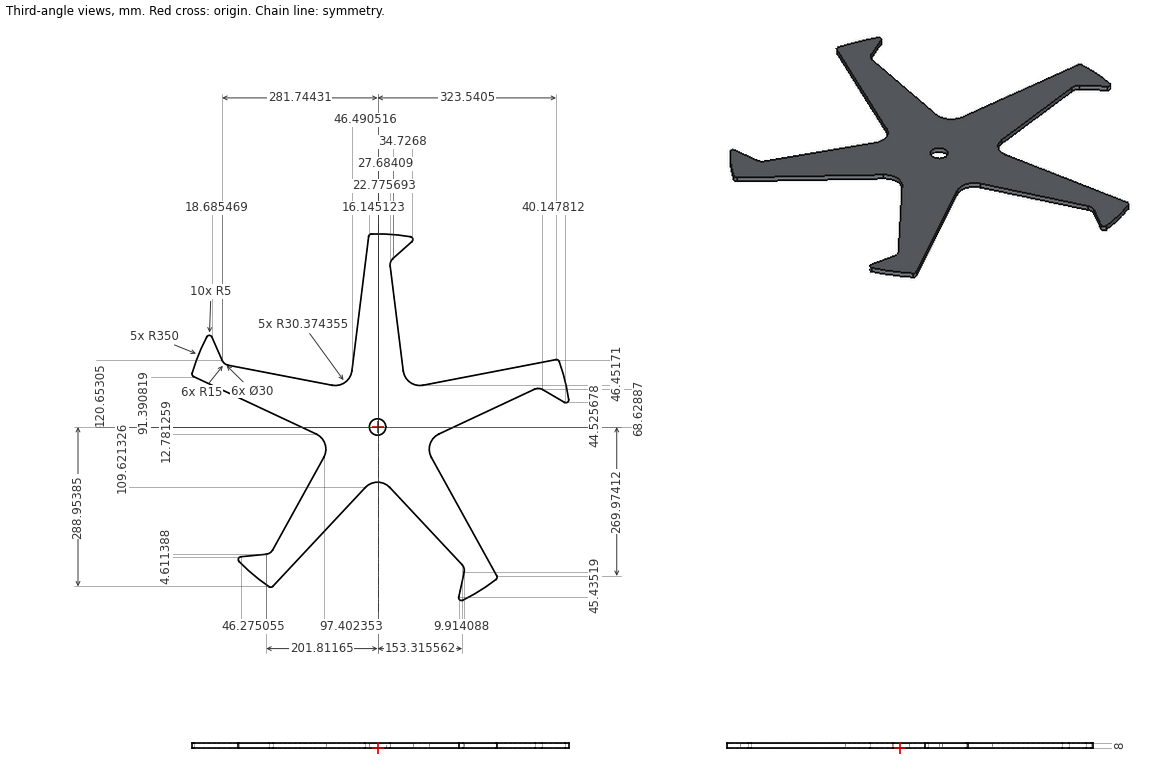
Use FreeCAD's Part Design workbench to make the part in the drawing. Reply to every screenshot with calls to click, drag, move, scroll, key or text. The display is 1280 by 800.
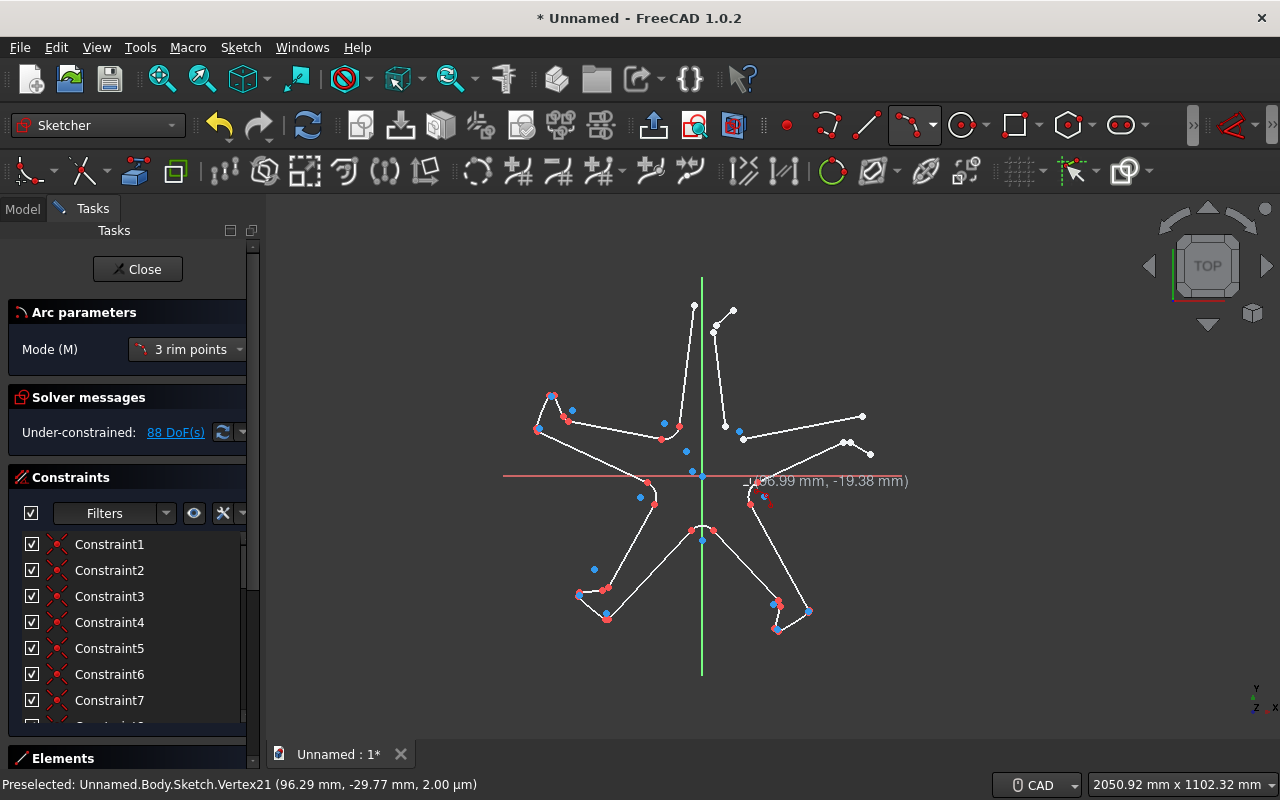
scroll(843, 442, up, 5)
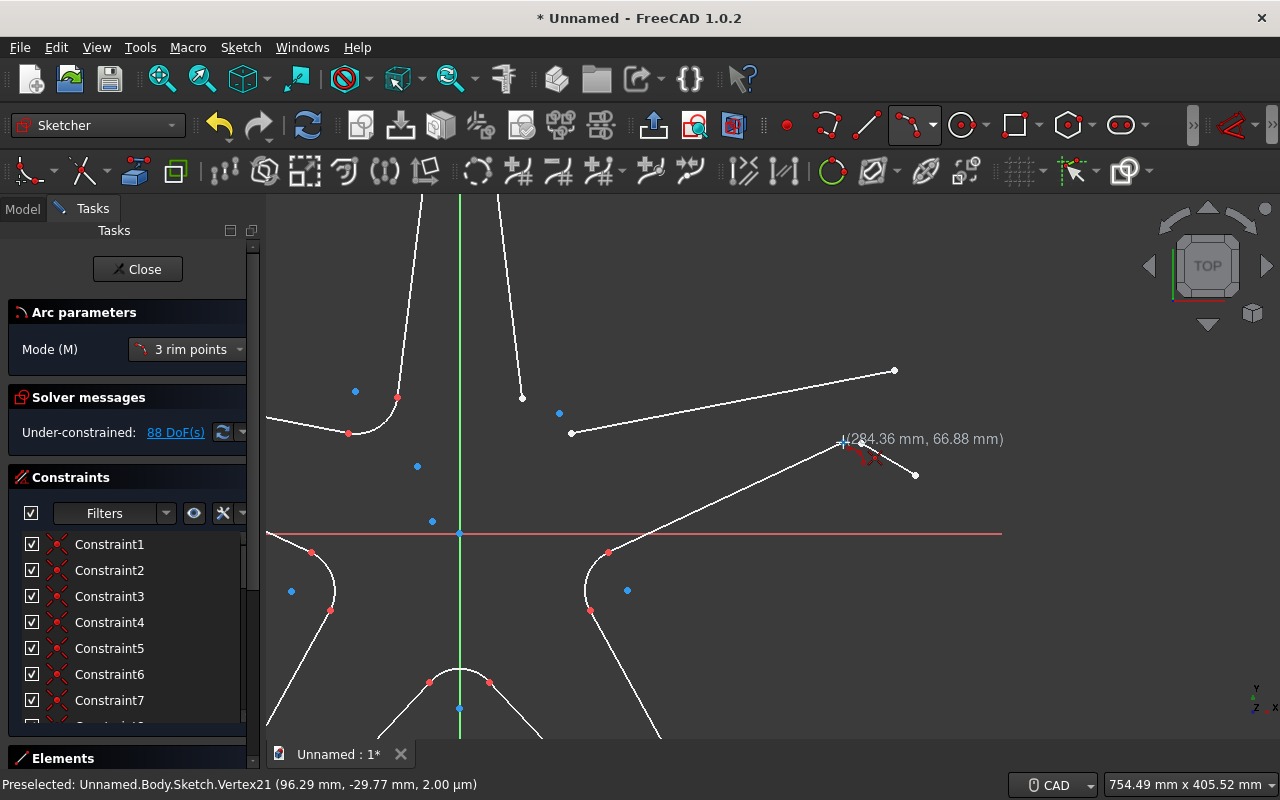
click(843, 442)
click(862, 443)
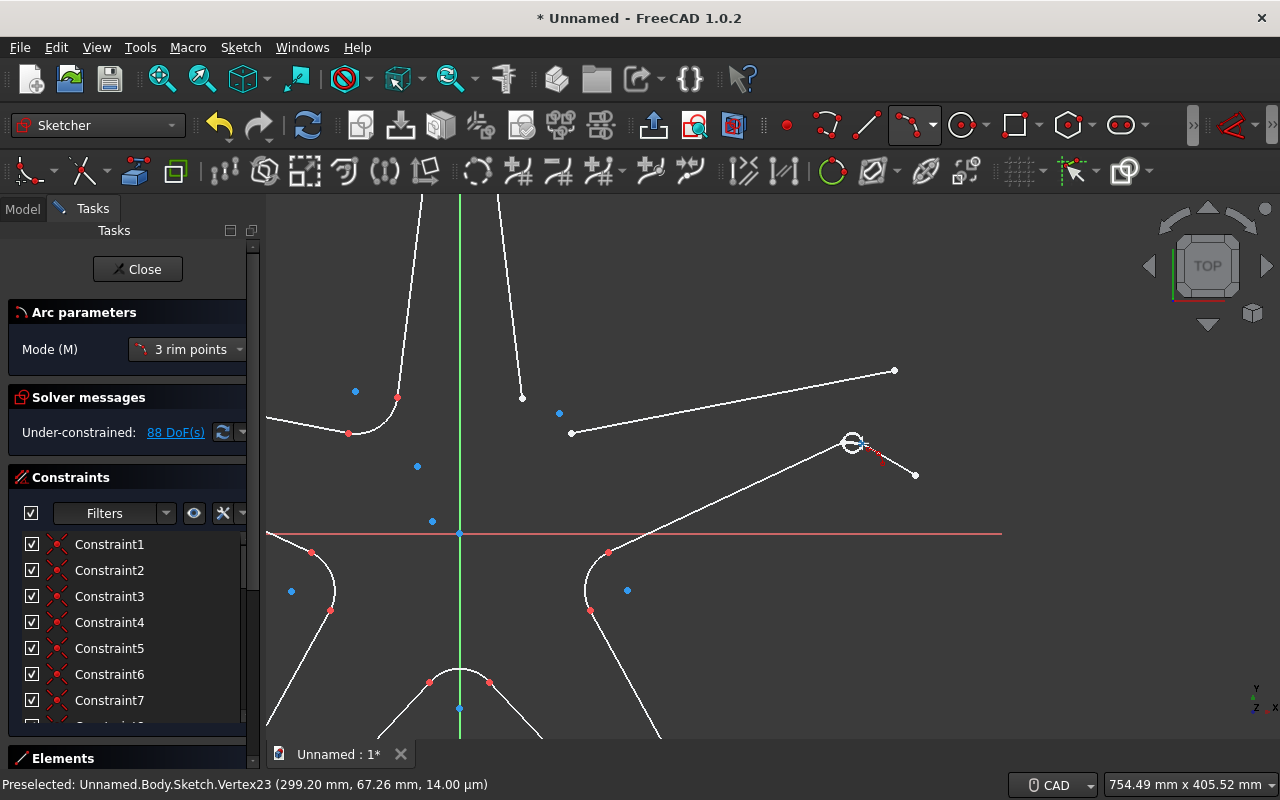
scroll(852, 440, up, 10)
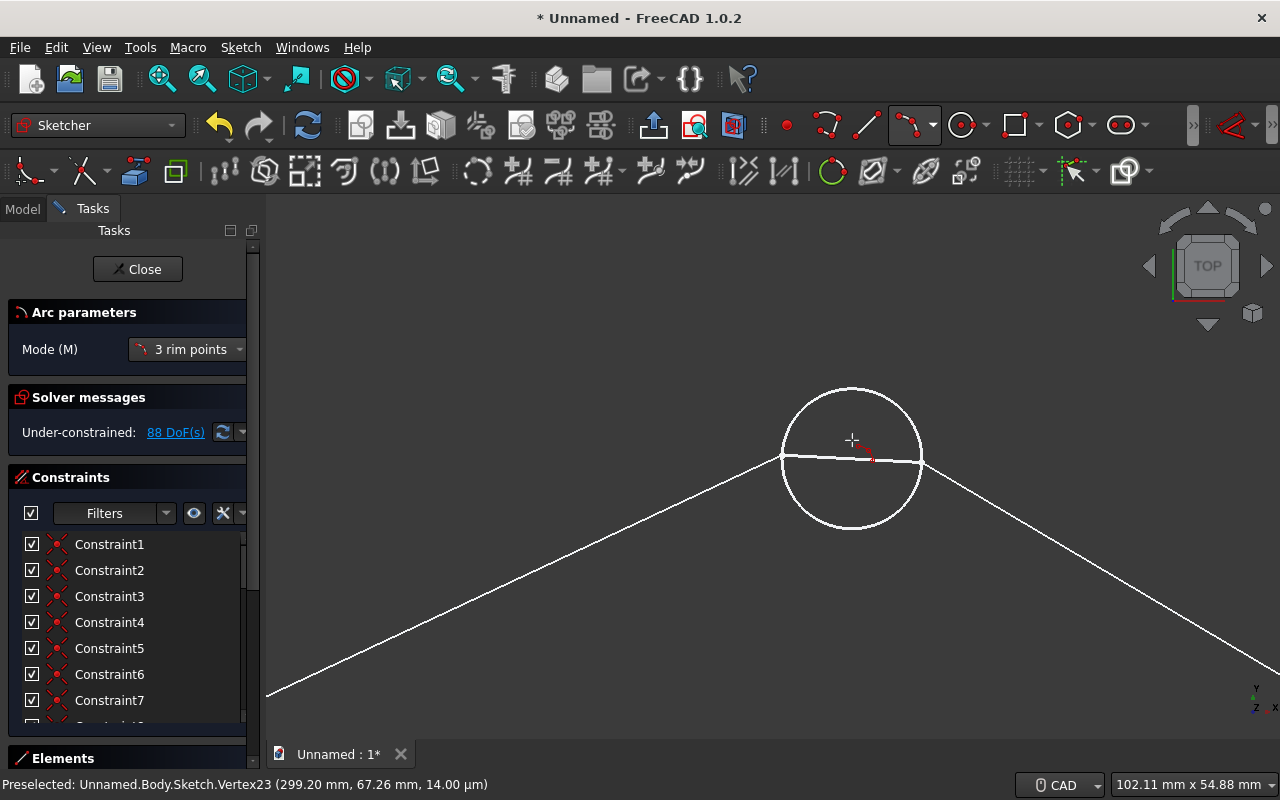
click(850, 435)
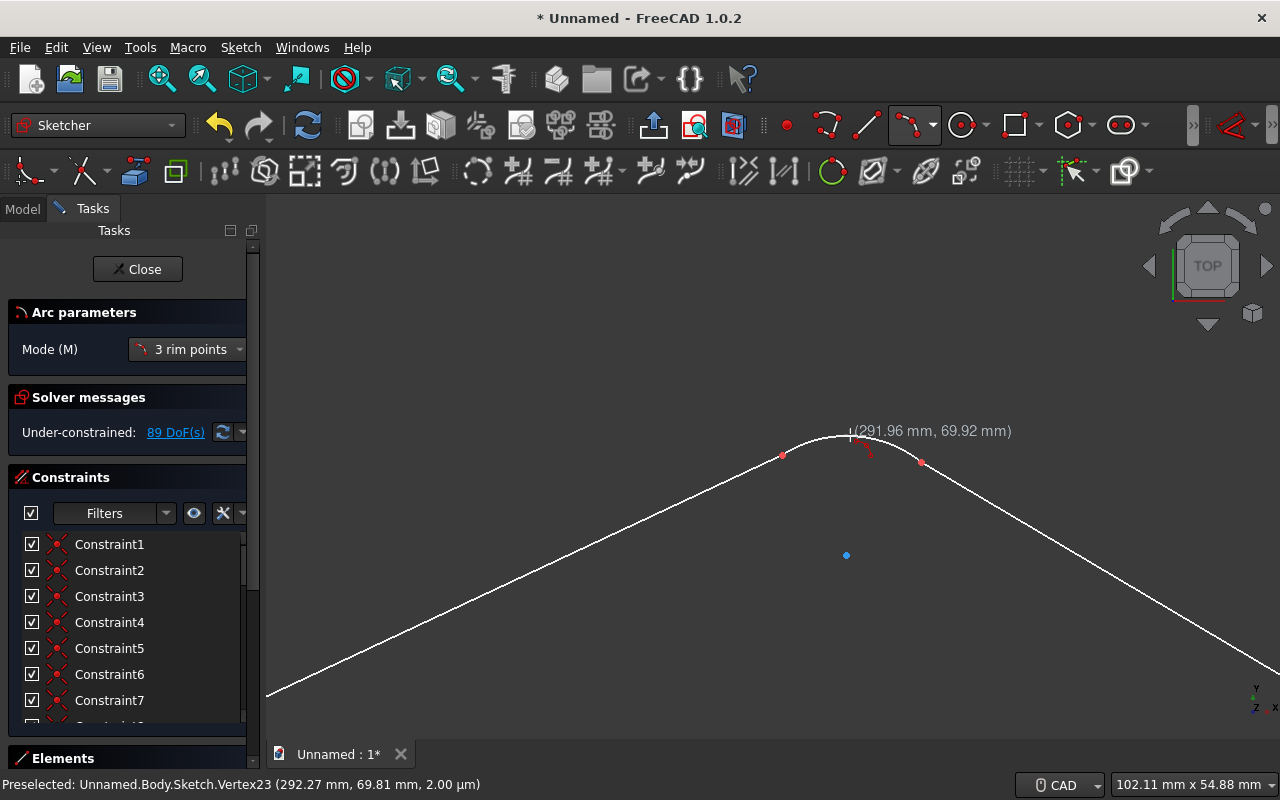
scroll(846, 441, down, 15)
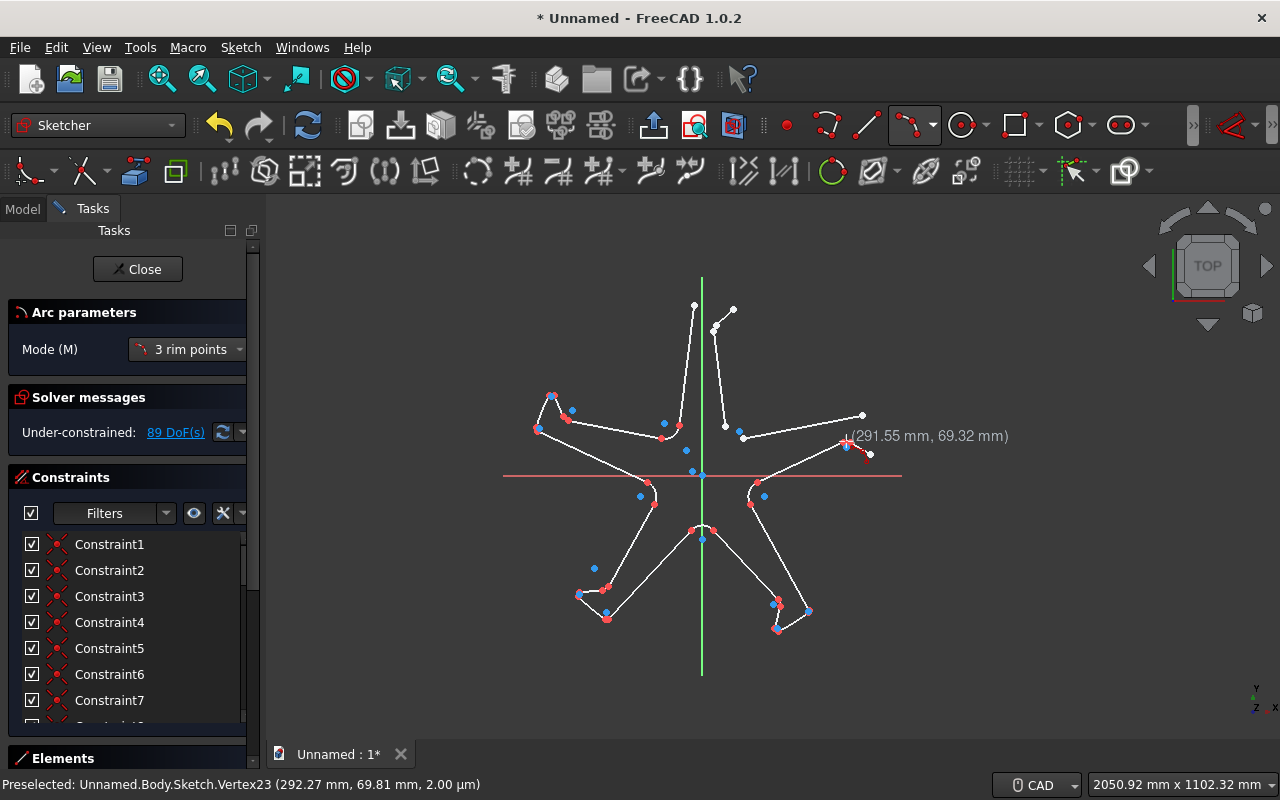
scroll(870, 454, up, 2)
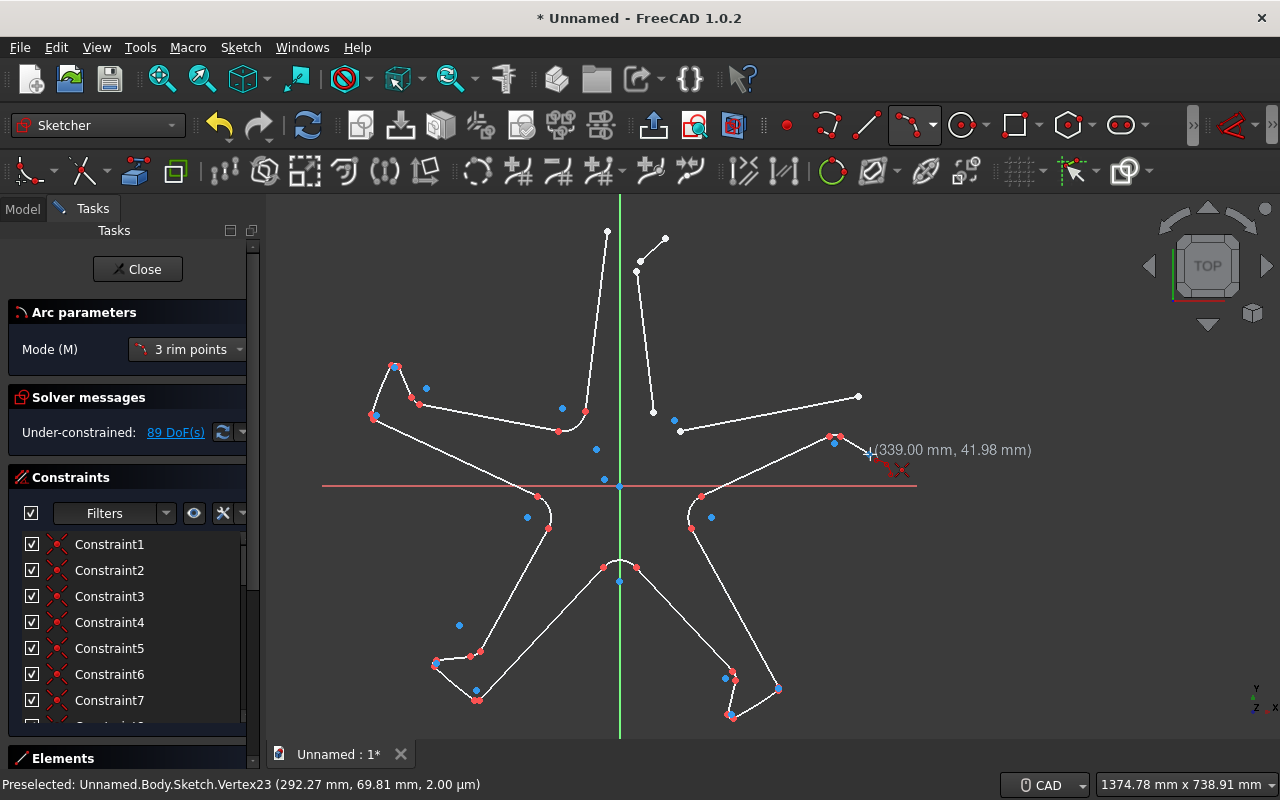
click(870, 454)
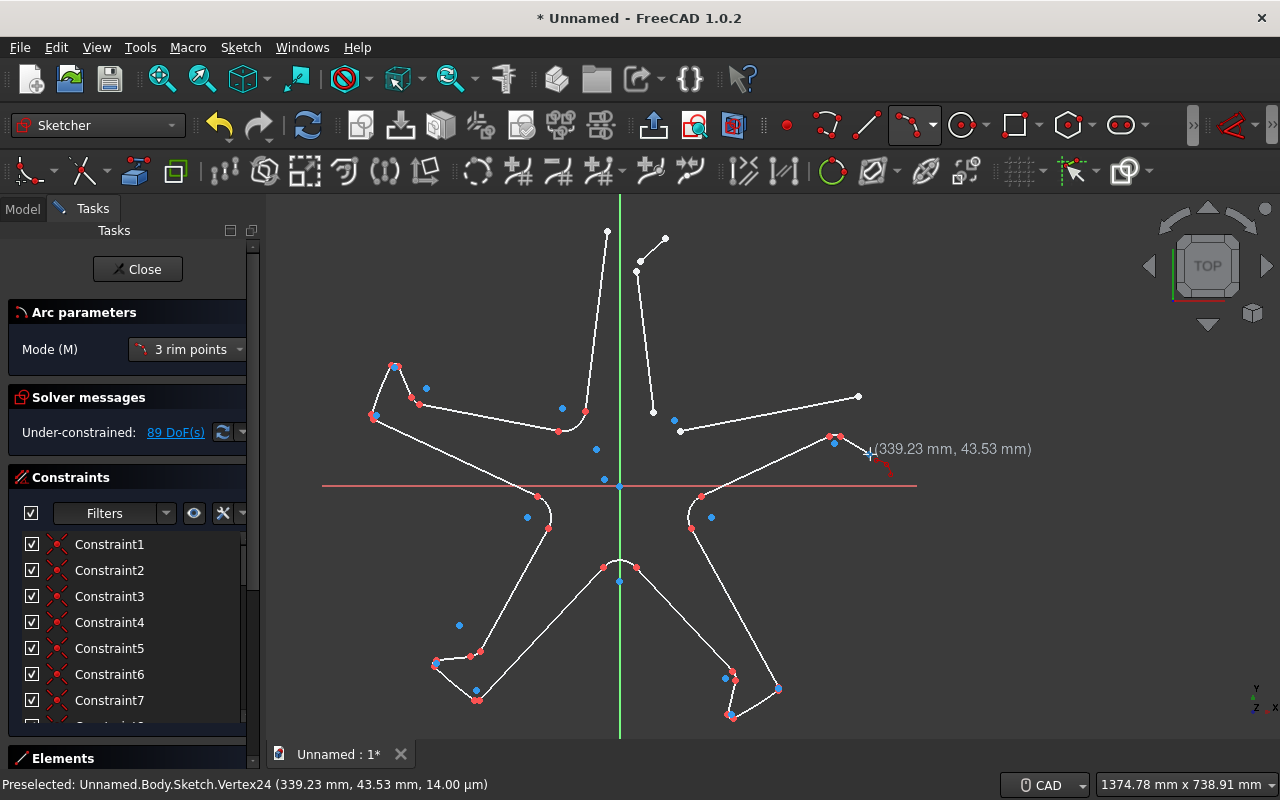
scroll(875, 450, up, 5)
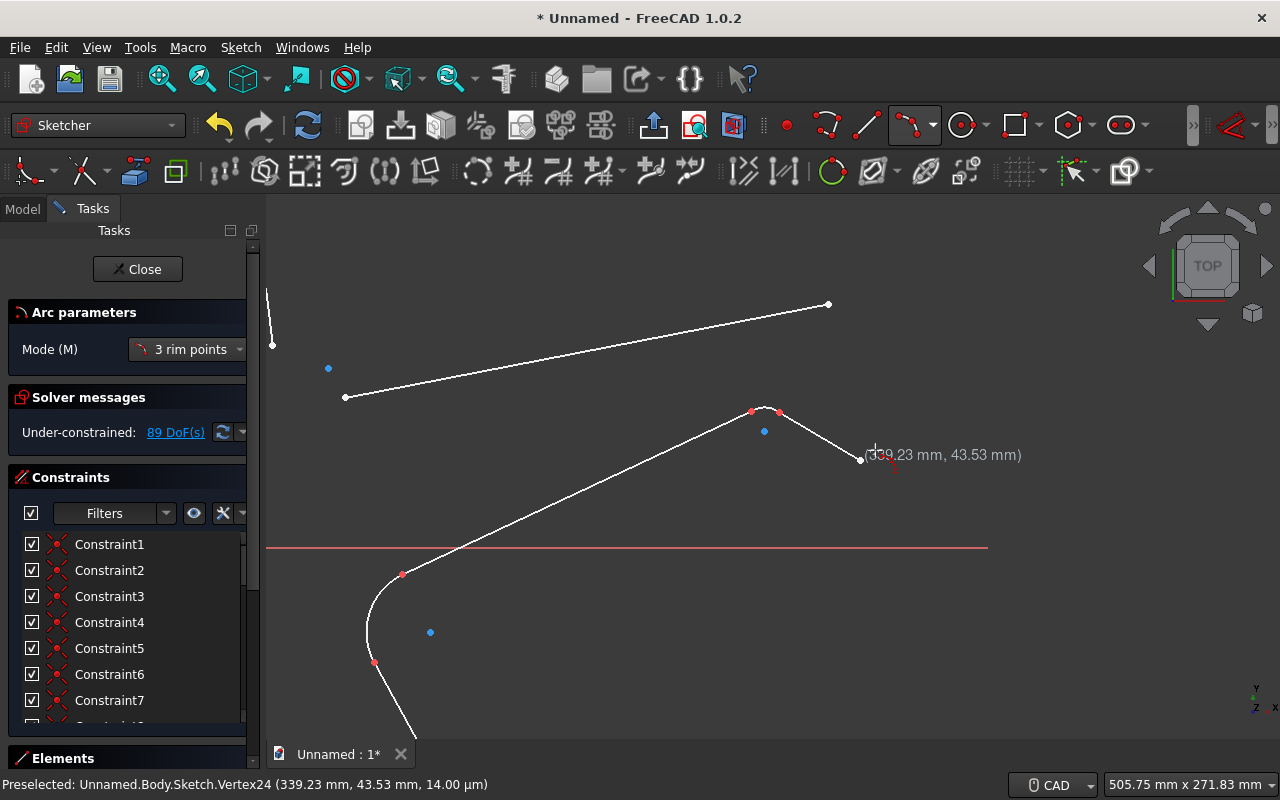
click(875, 448)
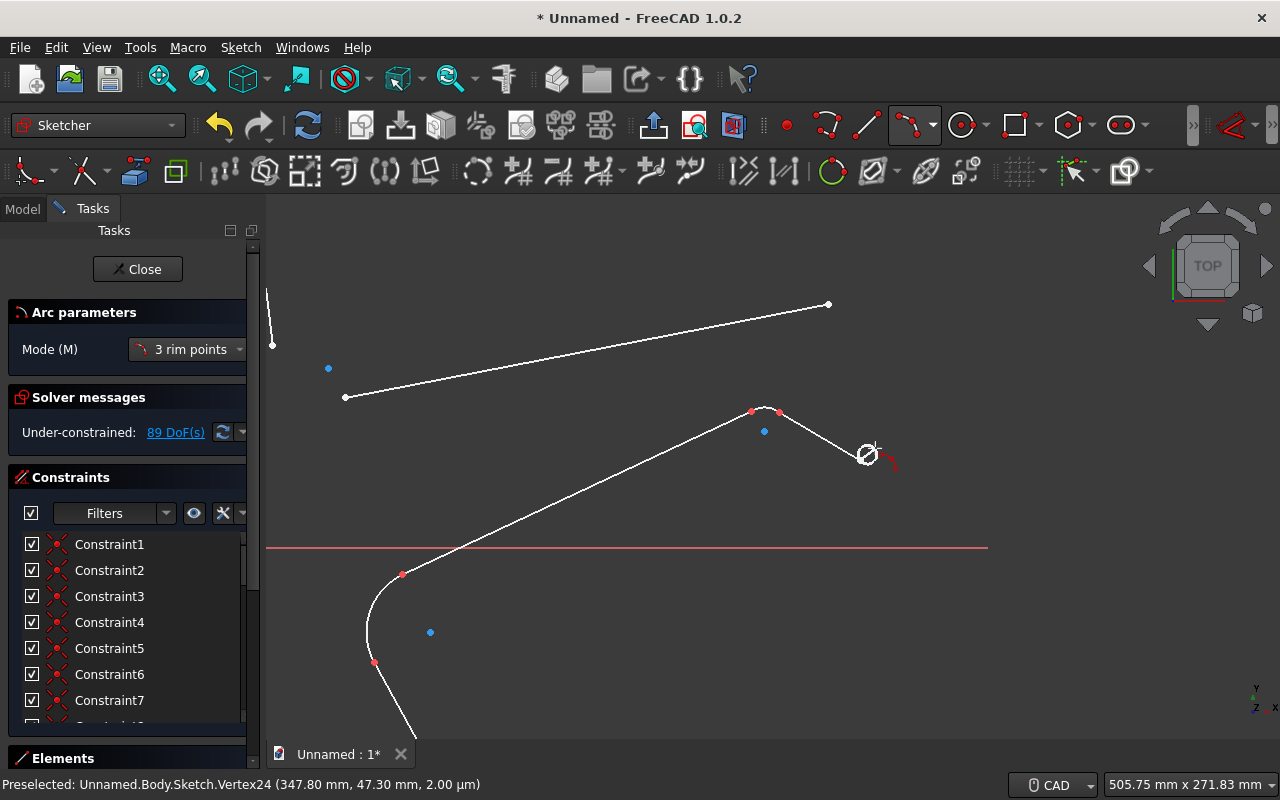
scroll(870, 458, up, 6)